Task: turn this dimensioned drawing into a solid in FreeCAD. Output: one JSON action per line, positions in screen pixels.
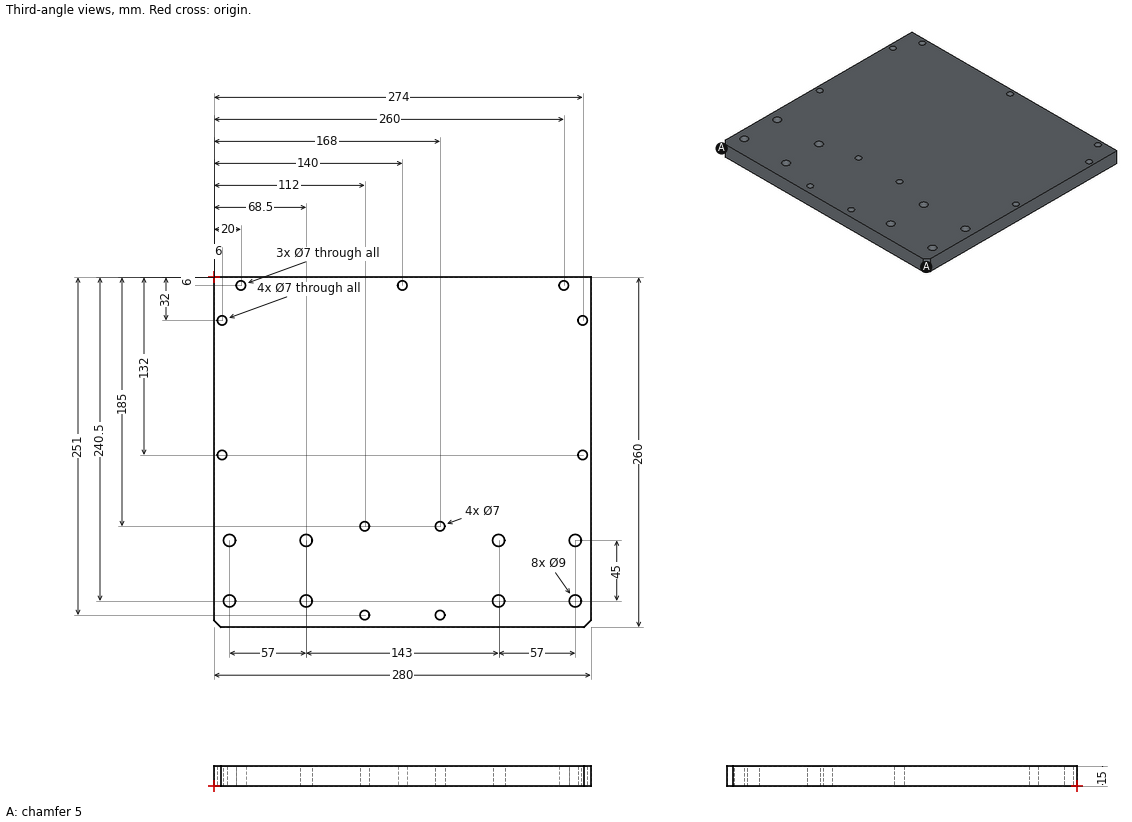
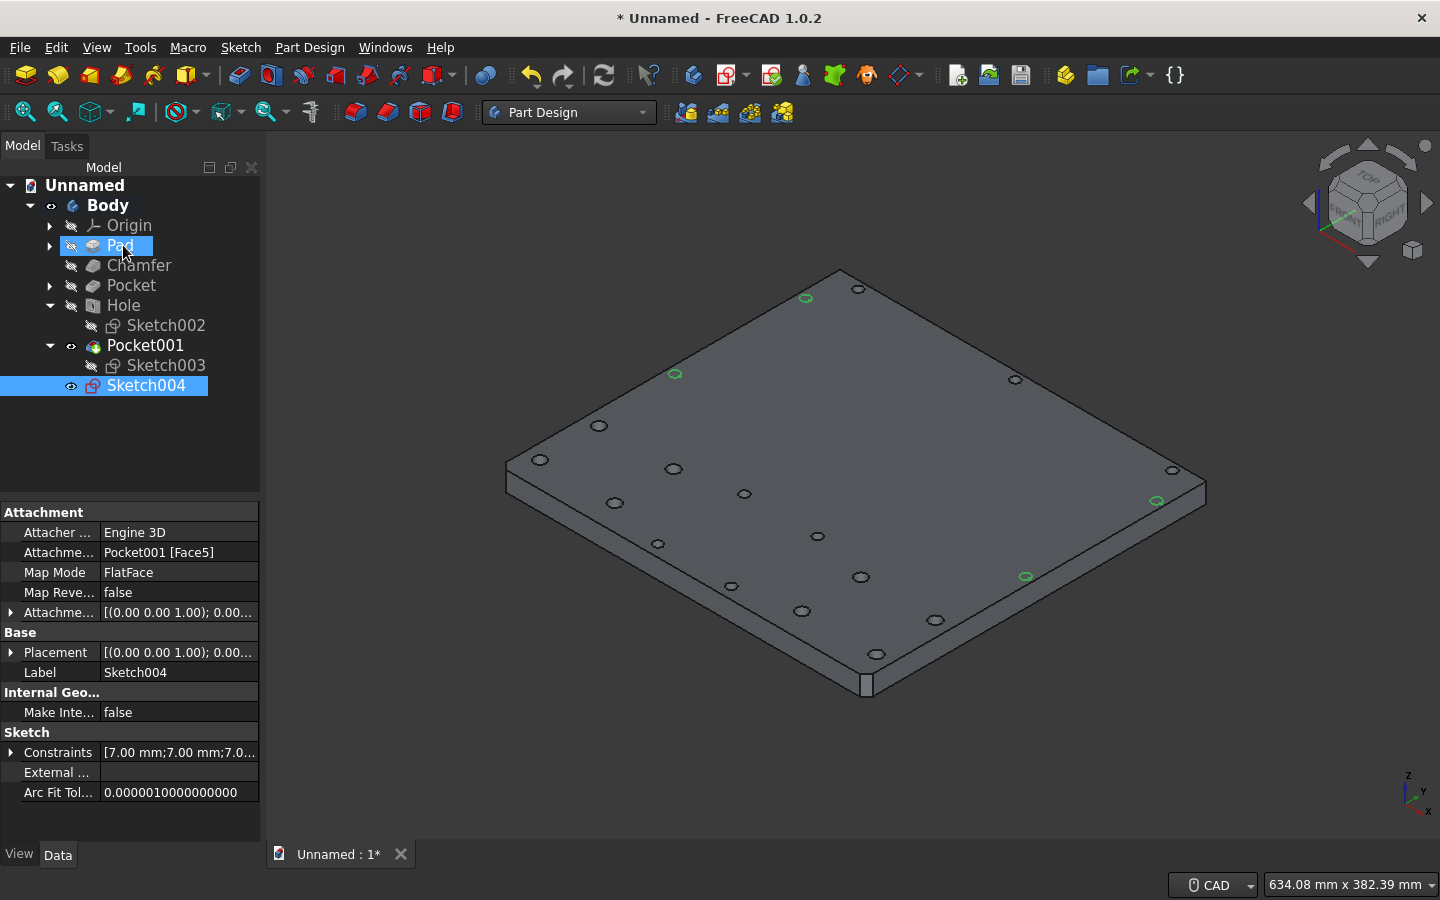
{"action": "left_click", "coordinate": [272, 76]}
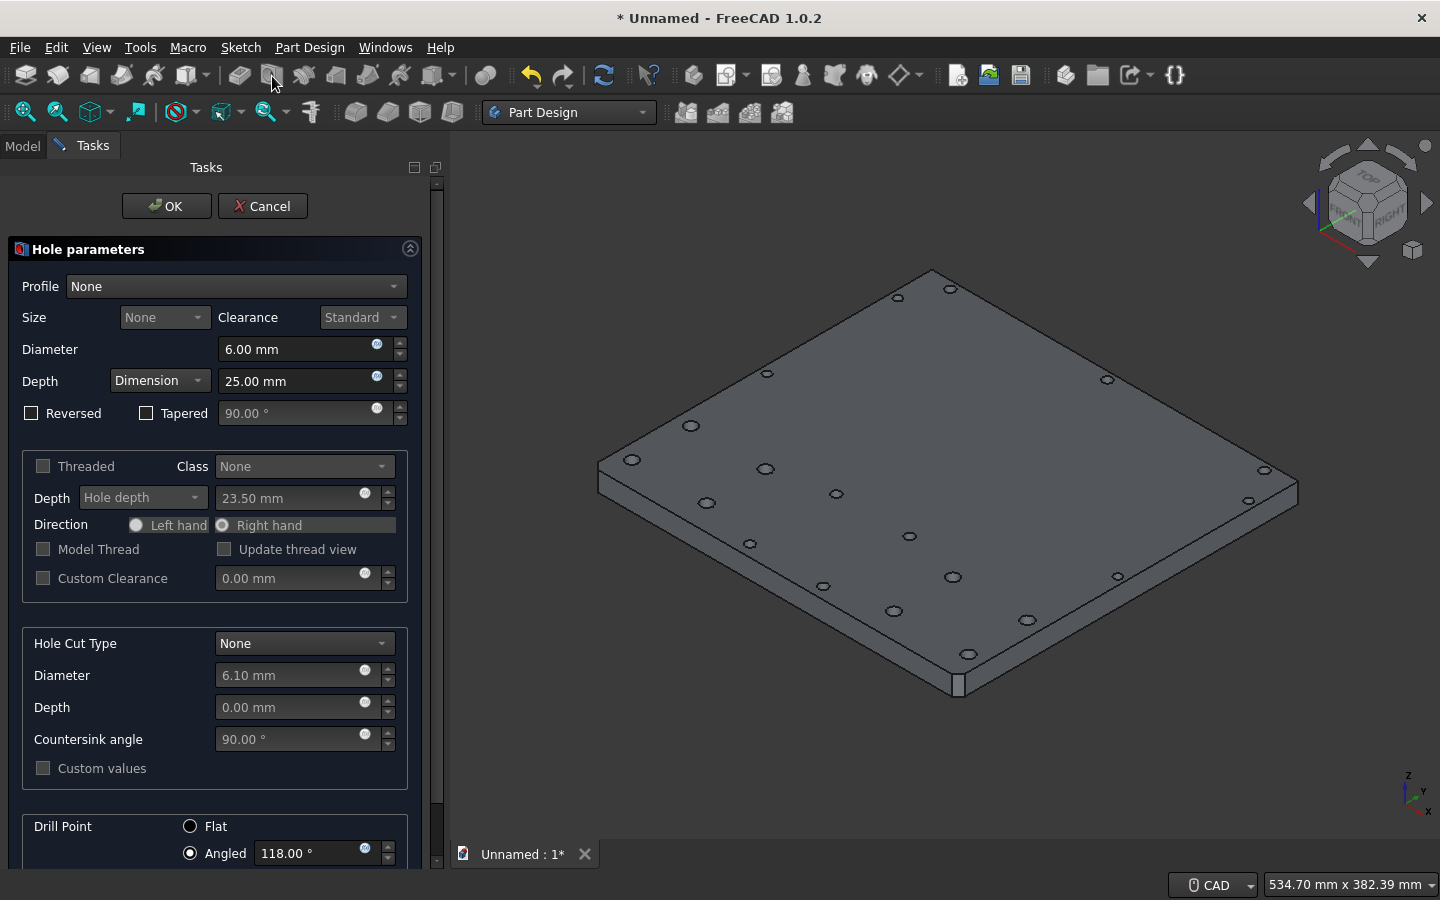
{"action": "triple_click", "coordinate": [305, 349]}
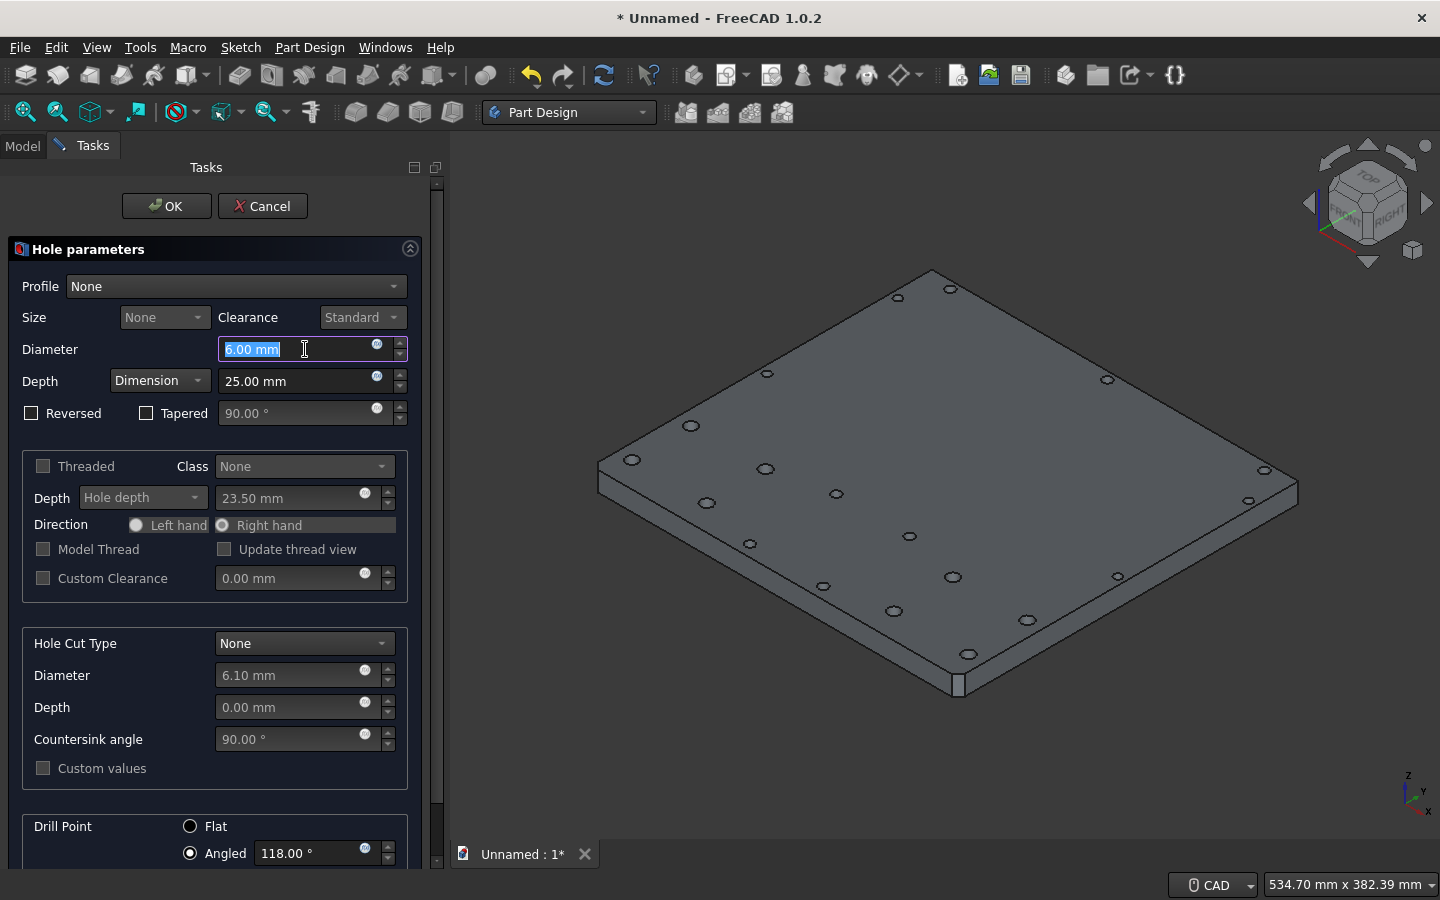
{"action": "type", "text": "7"}
{"action": "key", "text": "Tab"}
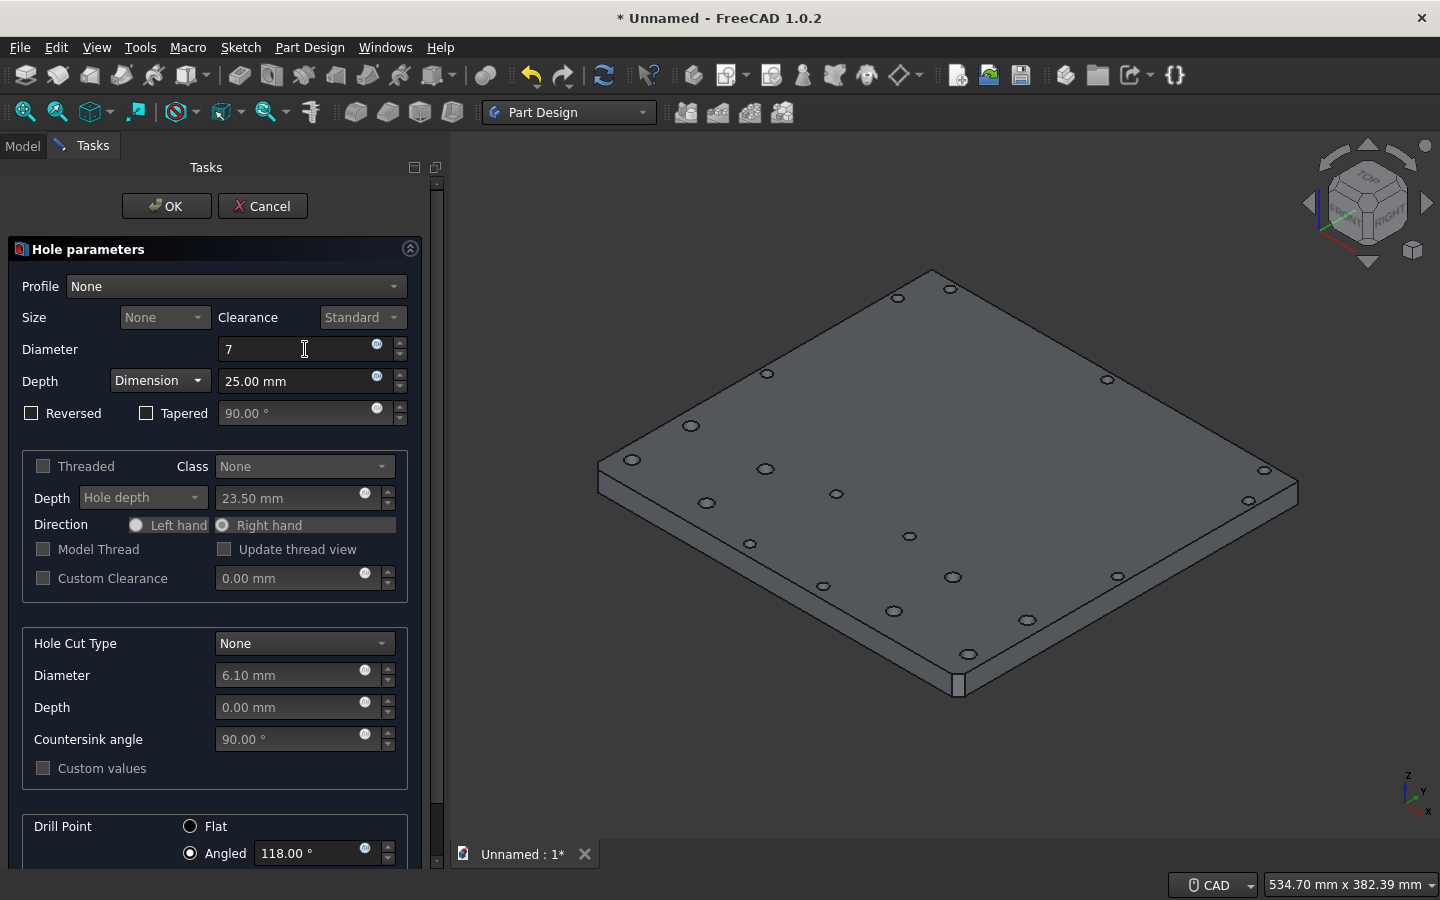
{"action": "left_click", "coordinate": [161, 380]}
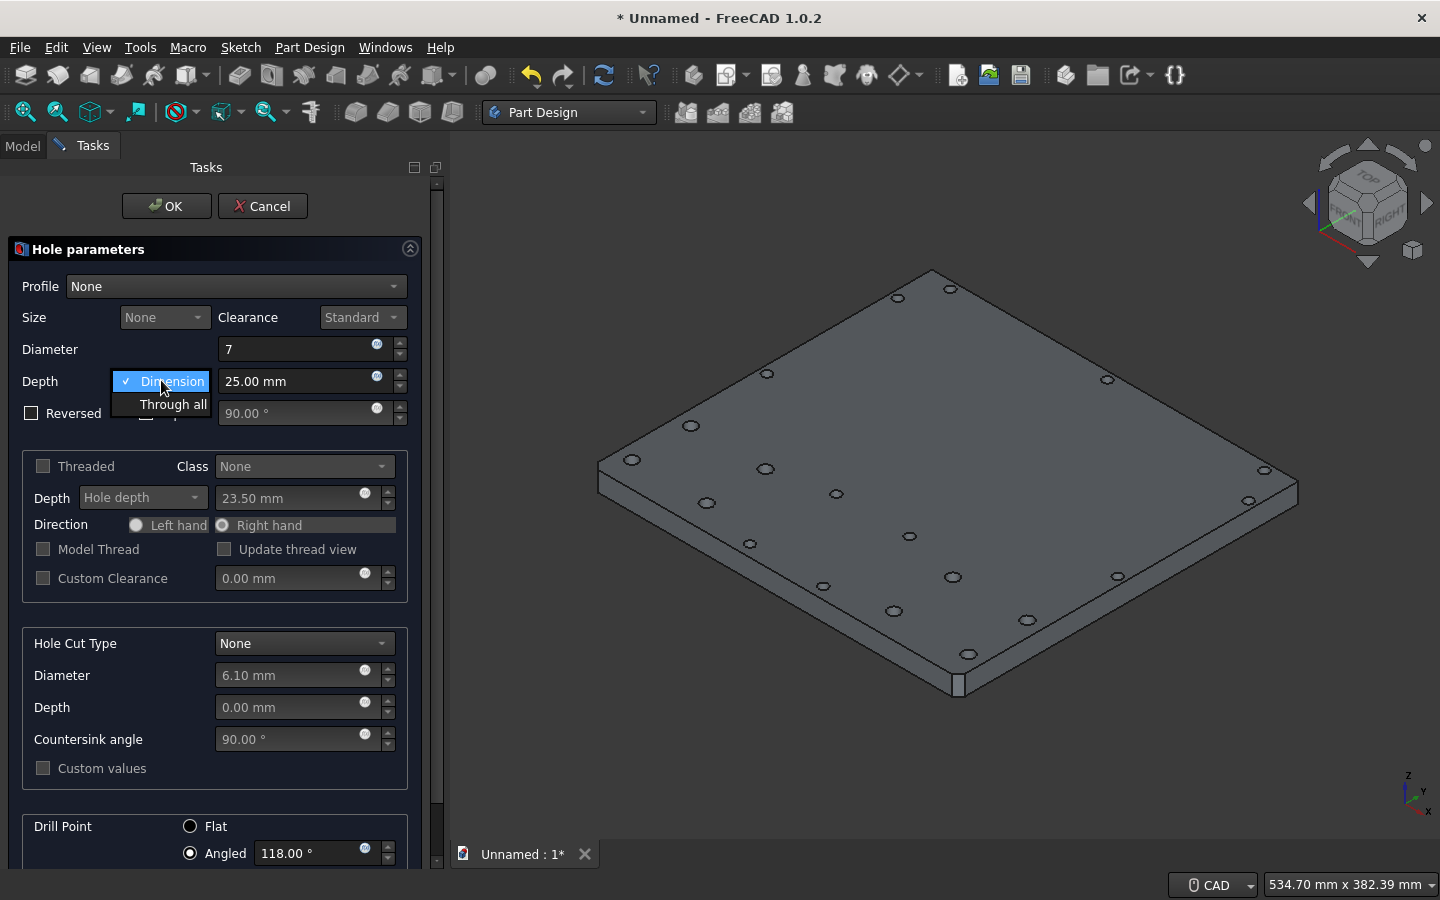
{"action": "left_click", "coordinate": [160, 404]}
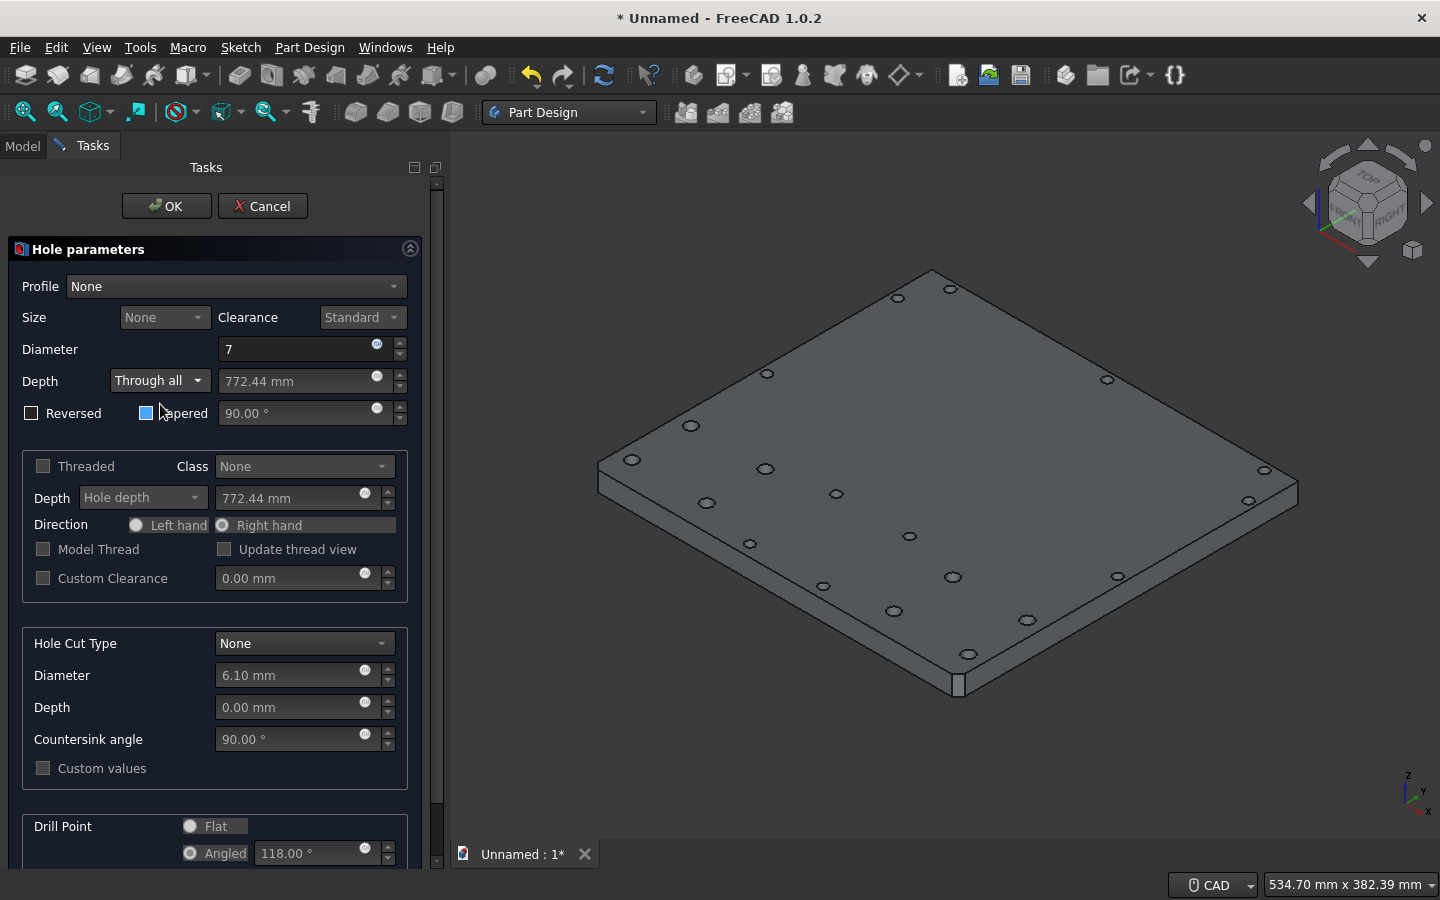
{"action": "left_click", "coordinate": [167, 206]}